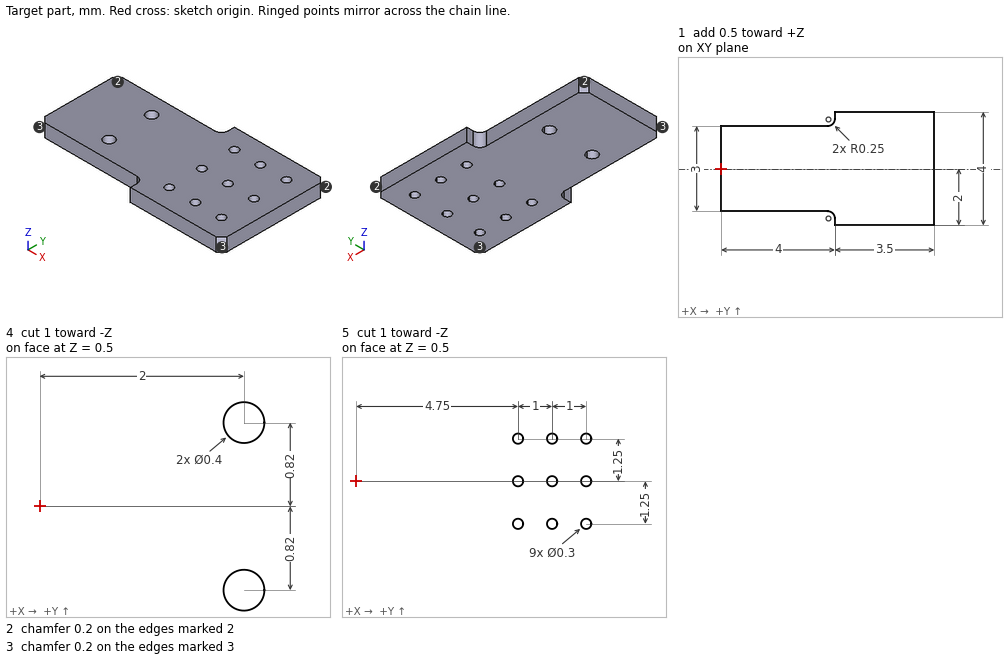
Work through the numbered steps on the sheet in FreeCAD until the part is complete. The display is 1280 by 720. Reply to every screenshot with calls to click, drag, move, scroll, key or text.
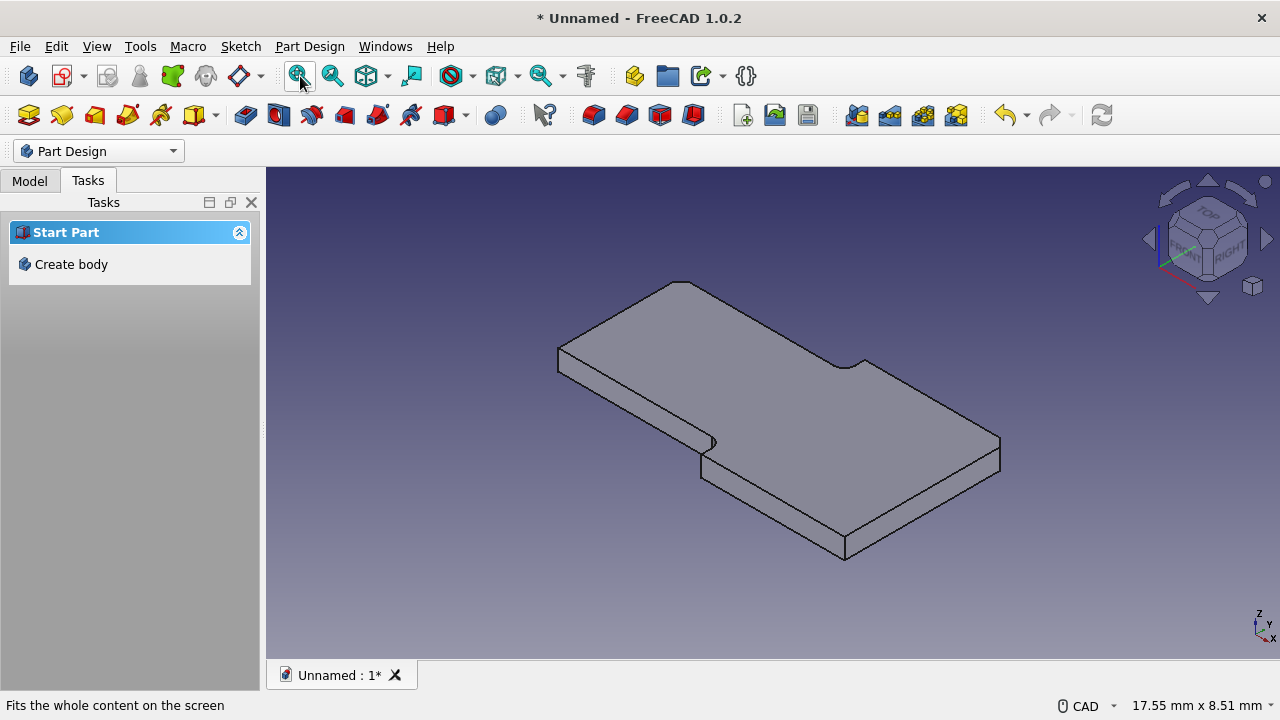
click(845, 548)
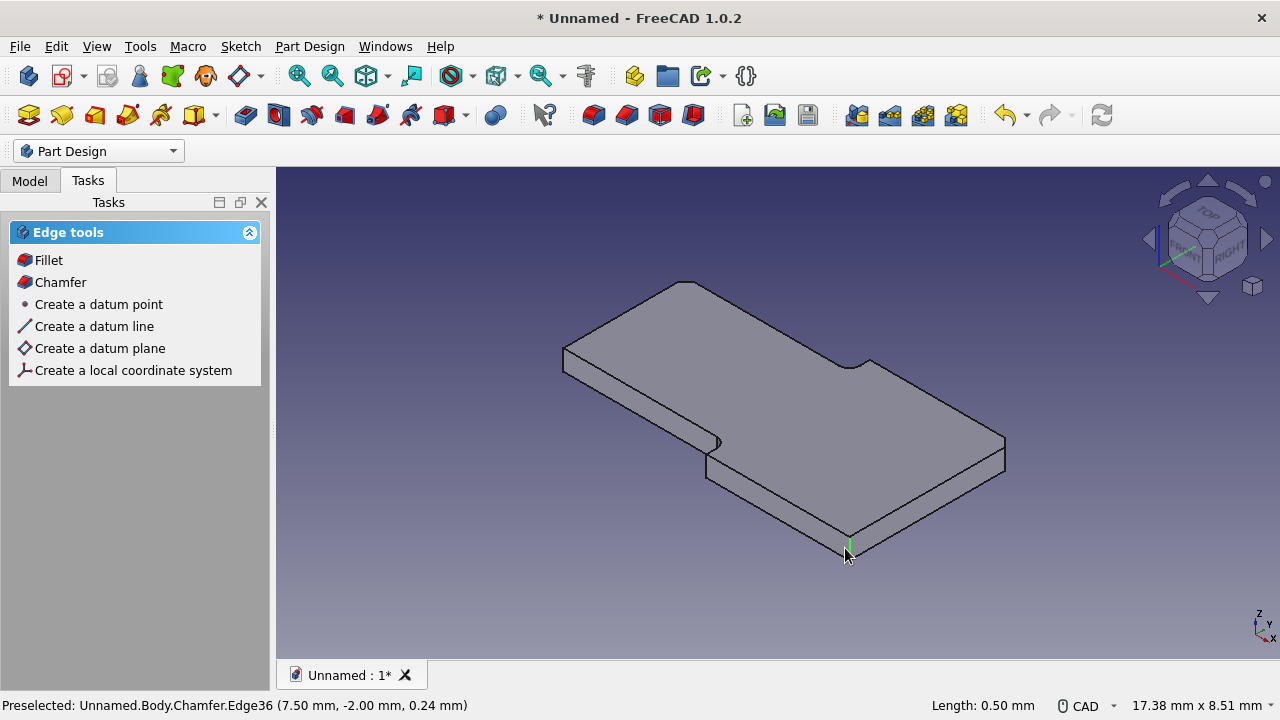
key(2)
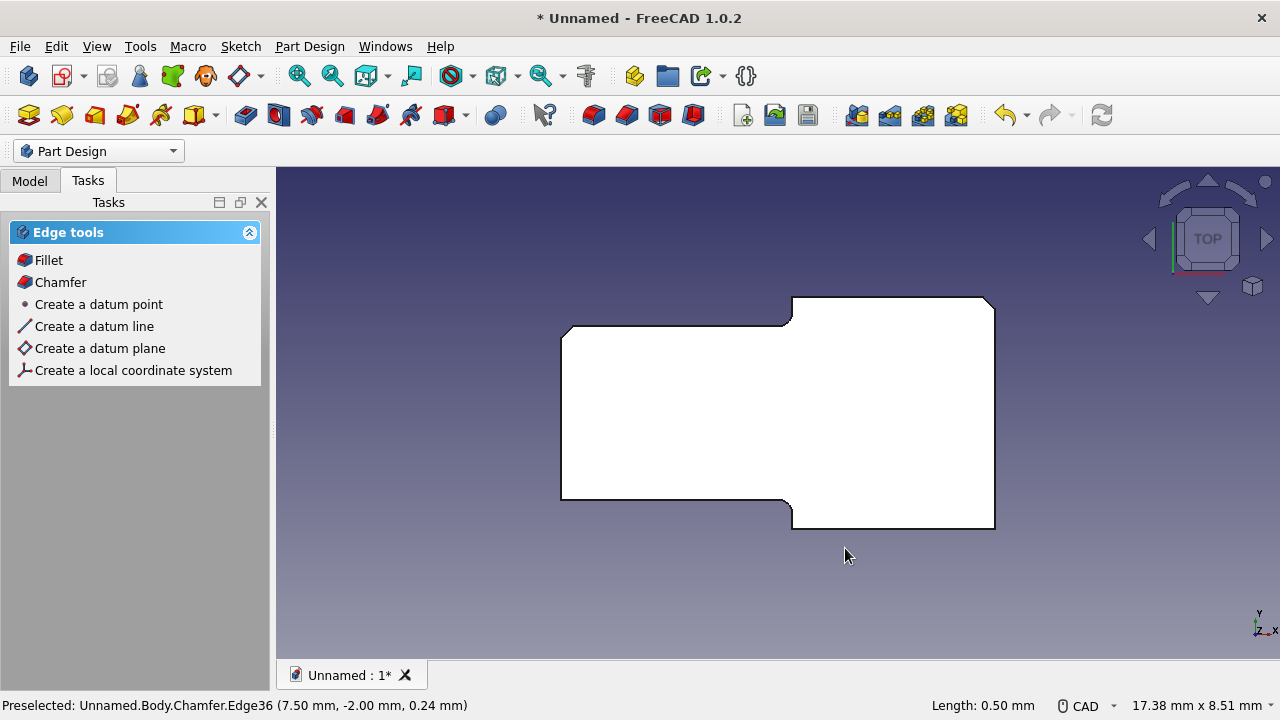
key(1)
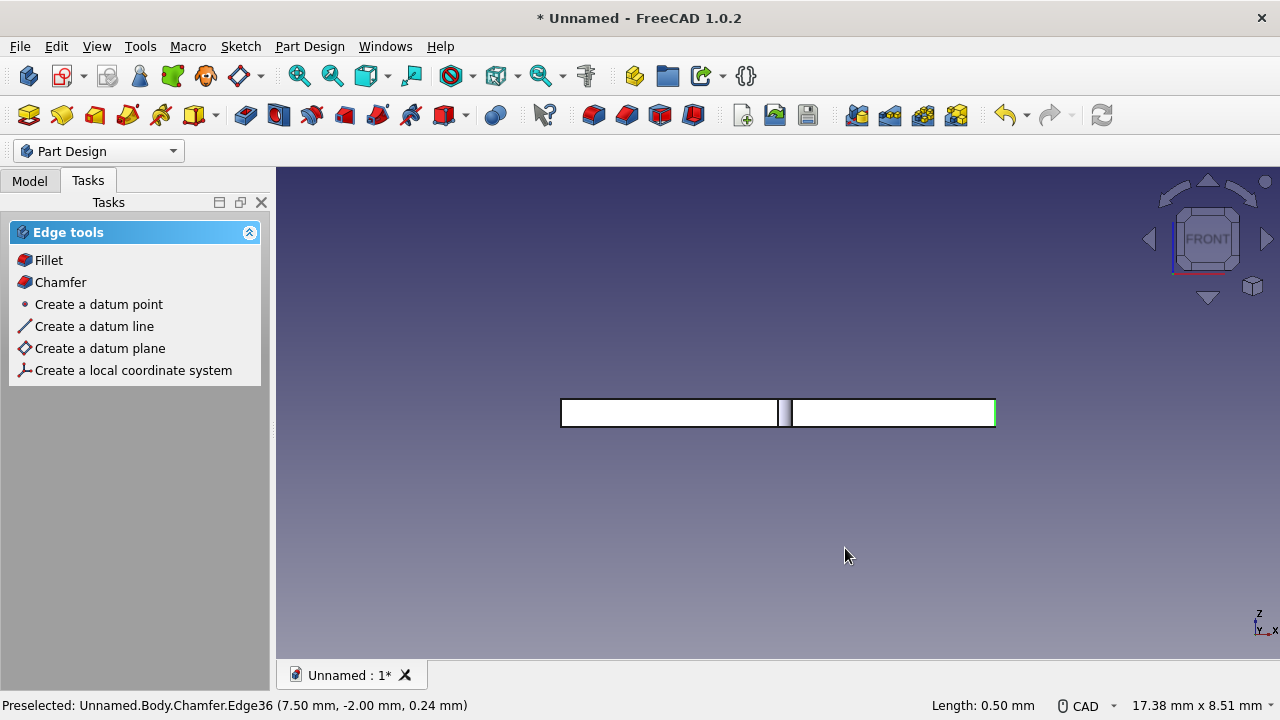
key(v)
key(f)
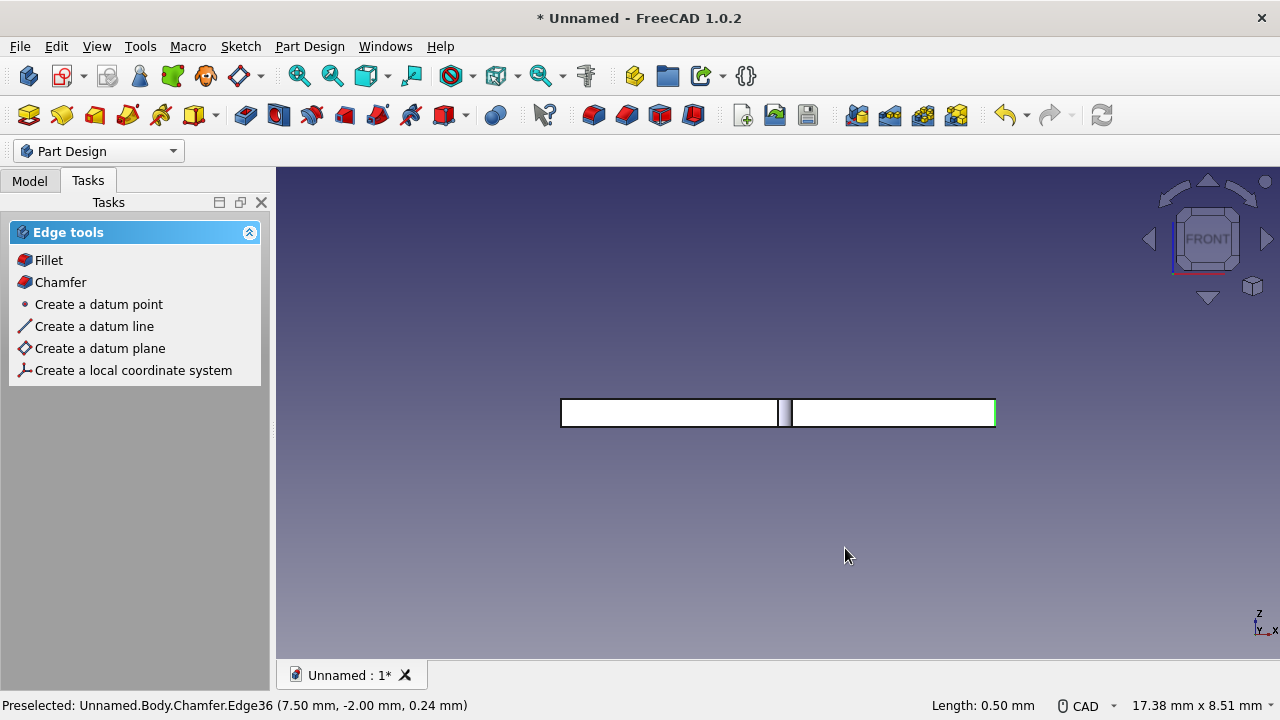
click(561, 412, ctrl)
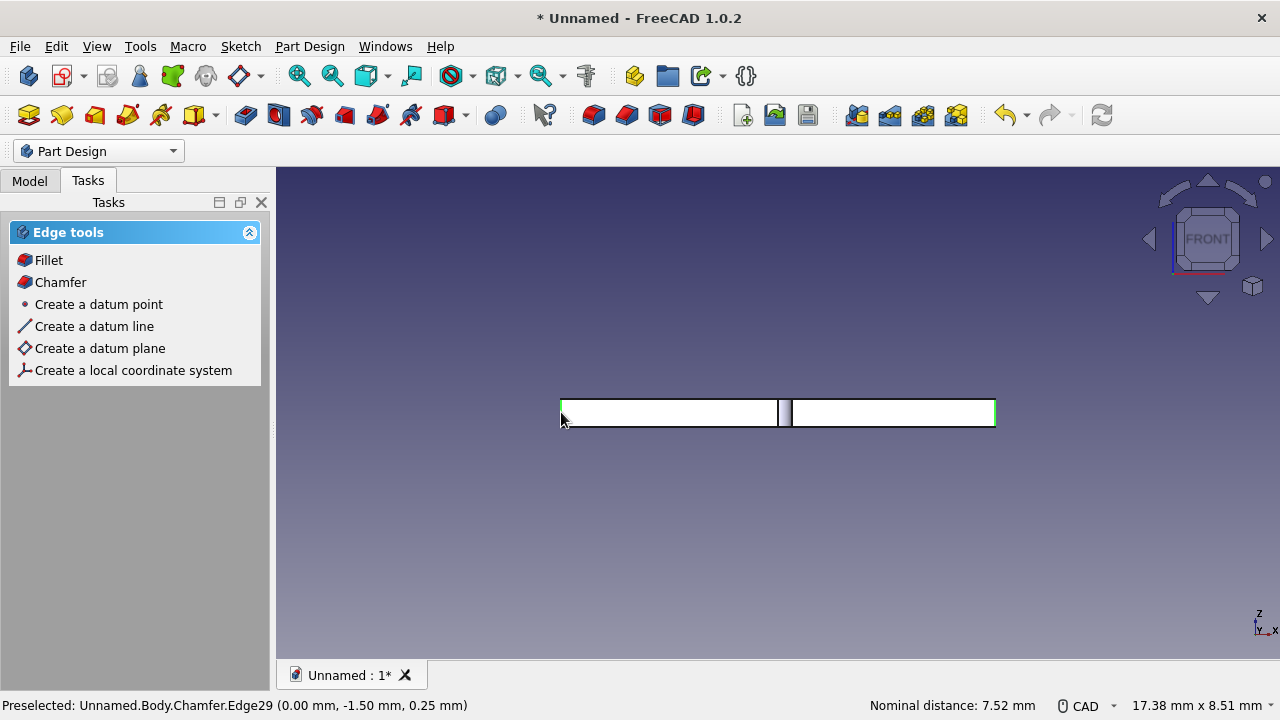
click(627, 116)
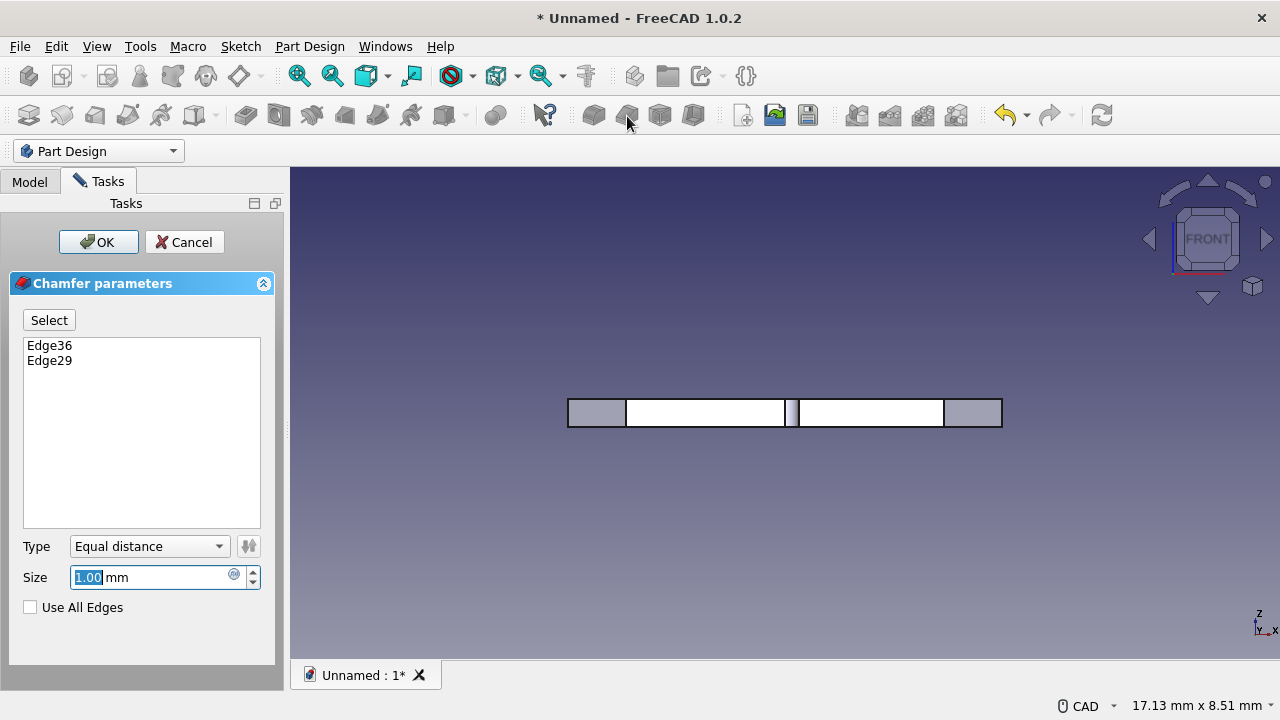
text(0.2)
key(Tab)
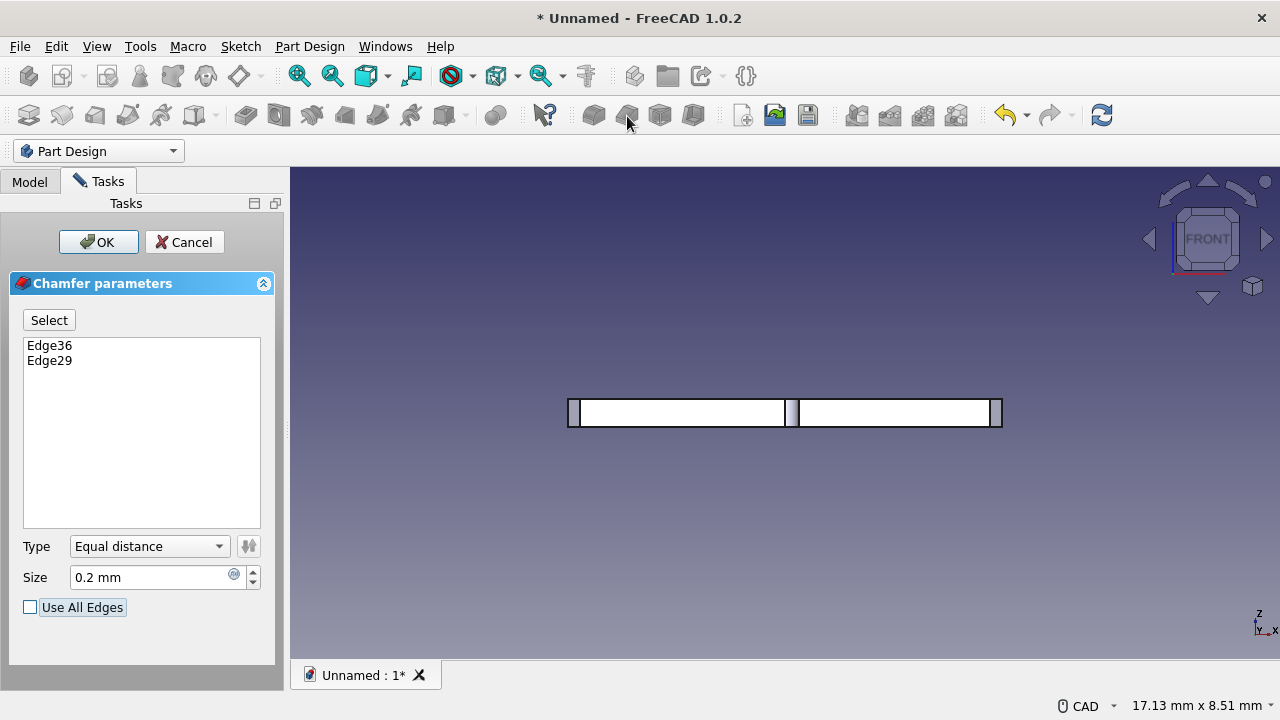
click(99, 242)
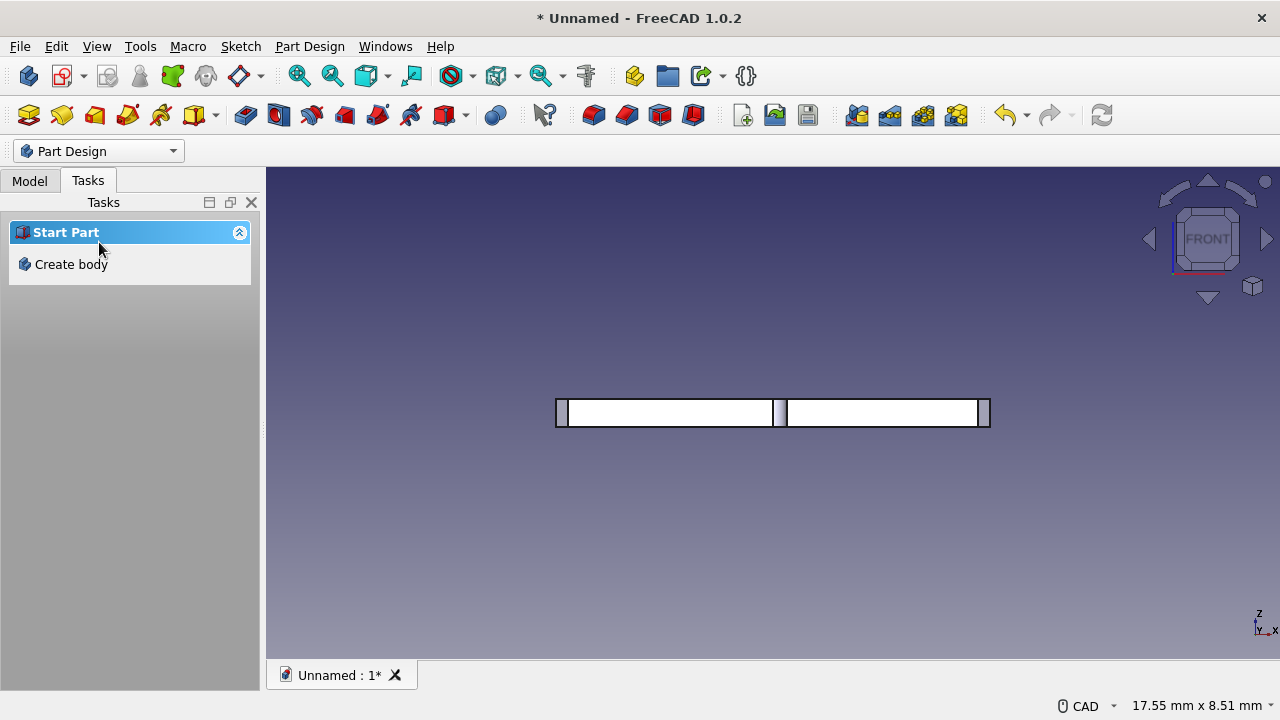
key(v)
key(f)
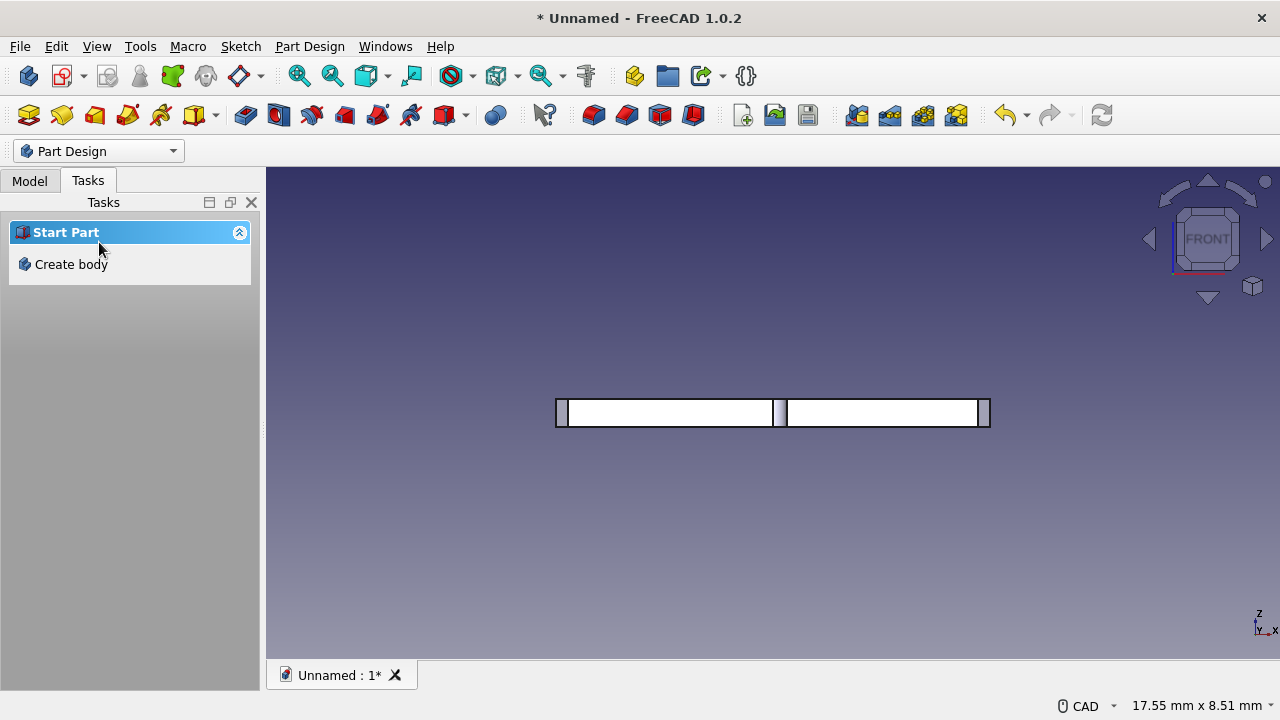
key(0)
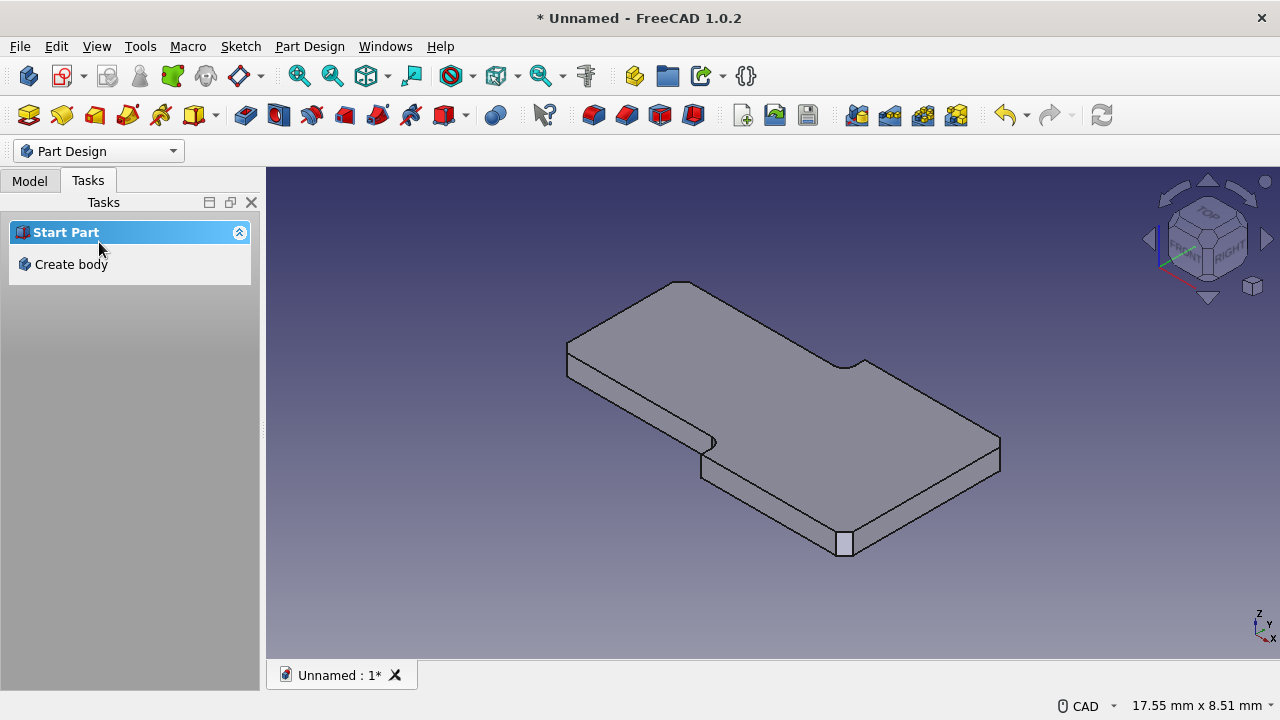
click(817, 425)